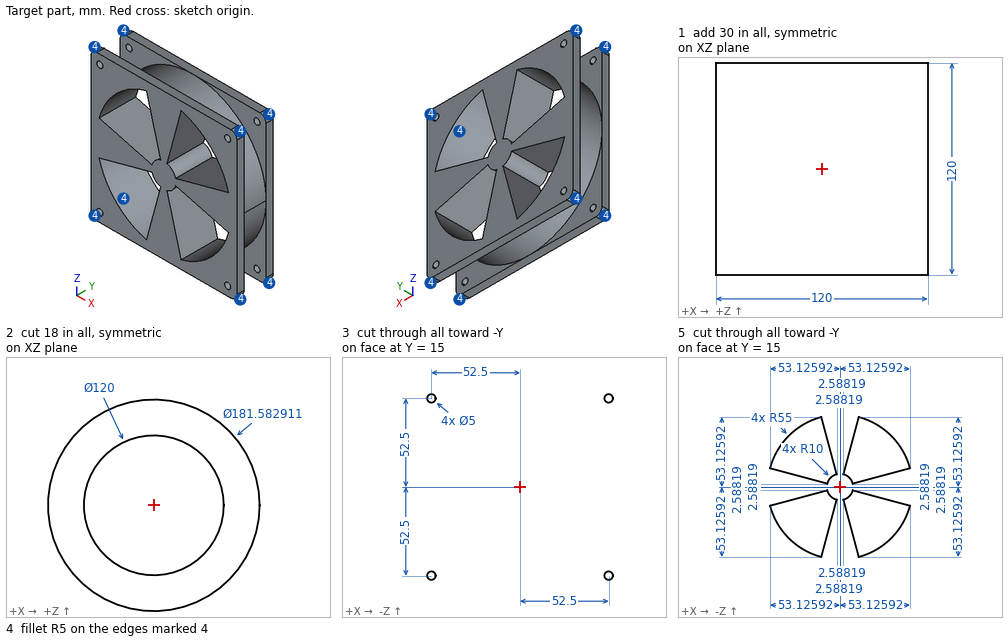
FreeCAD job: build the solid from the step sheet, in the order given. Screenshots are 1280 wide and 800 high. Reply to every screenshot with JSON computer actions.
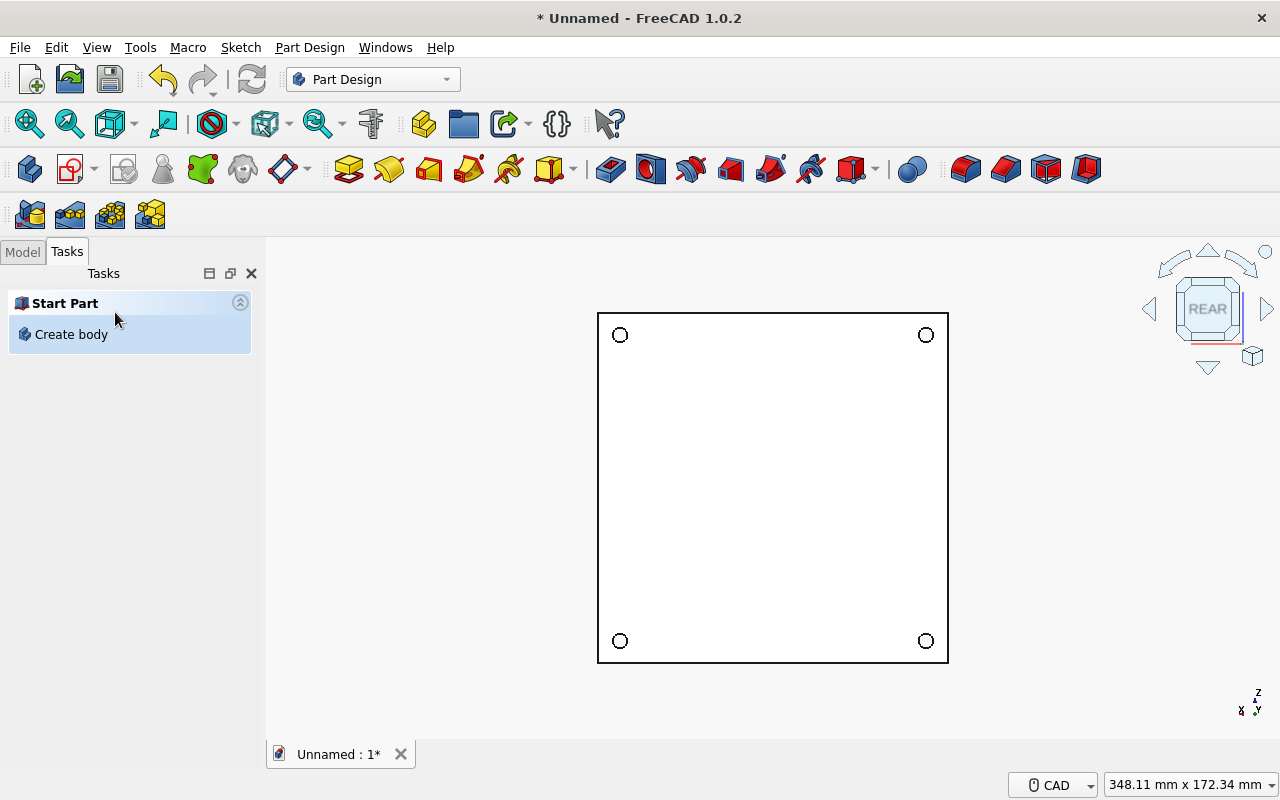
{"action": "scroll", "coordinate": [598, 312], "scroll_direction": "up", "scroll_amount": 5}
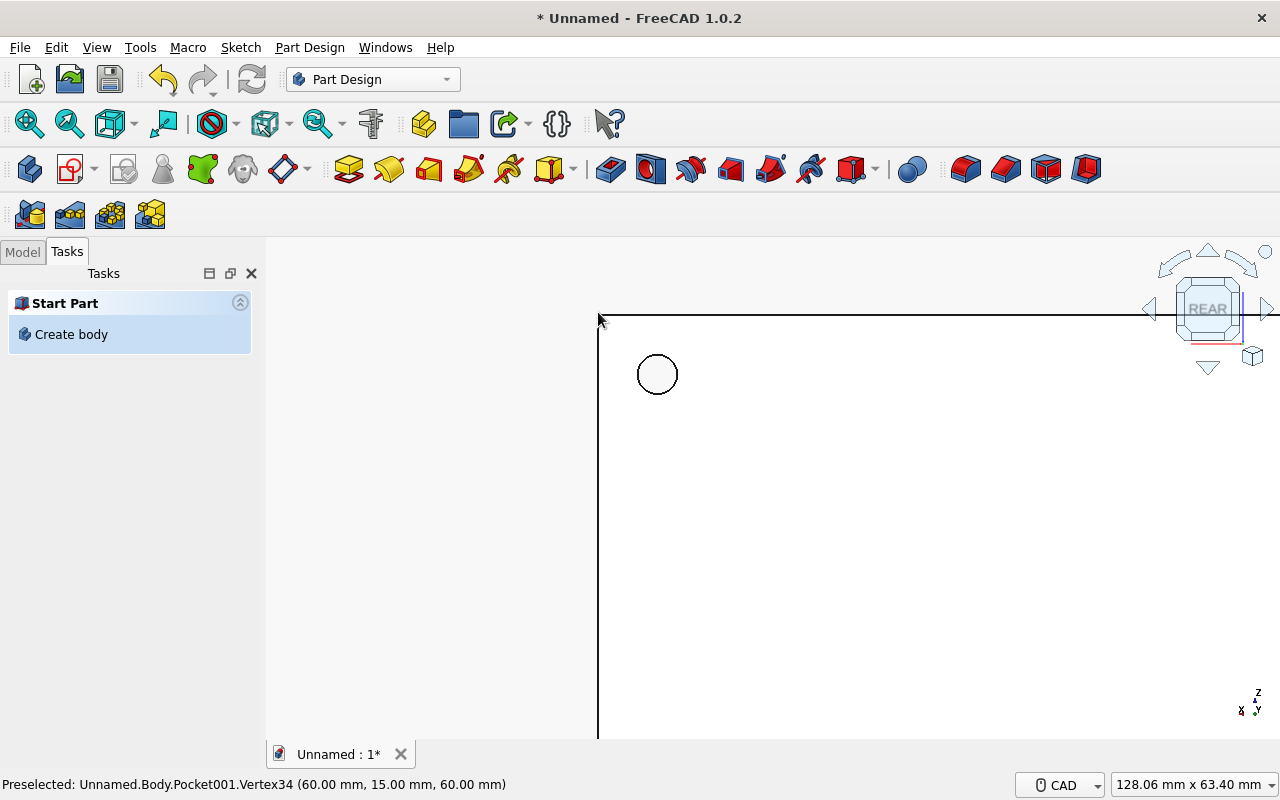
{"action": "left_click", "coordinate": [30, 124]}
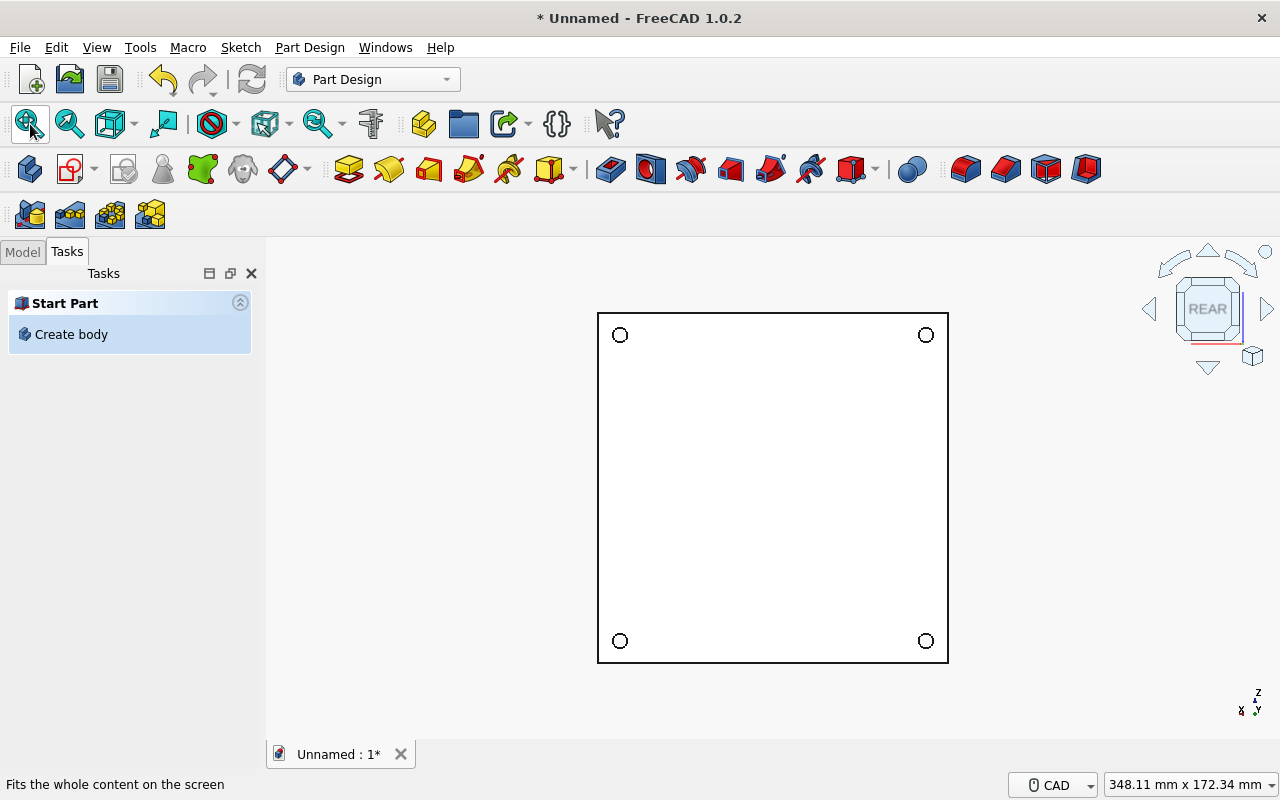
{"action": "key", "text": "0"}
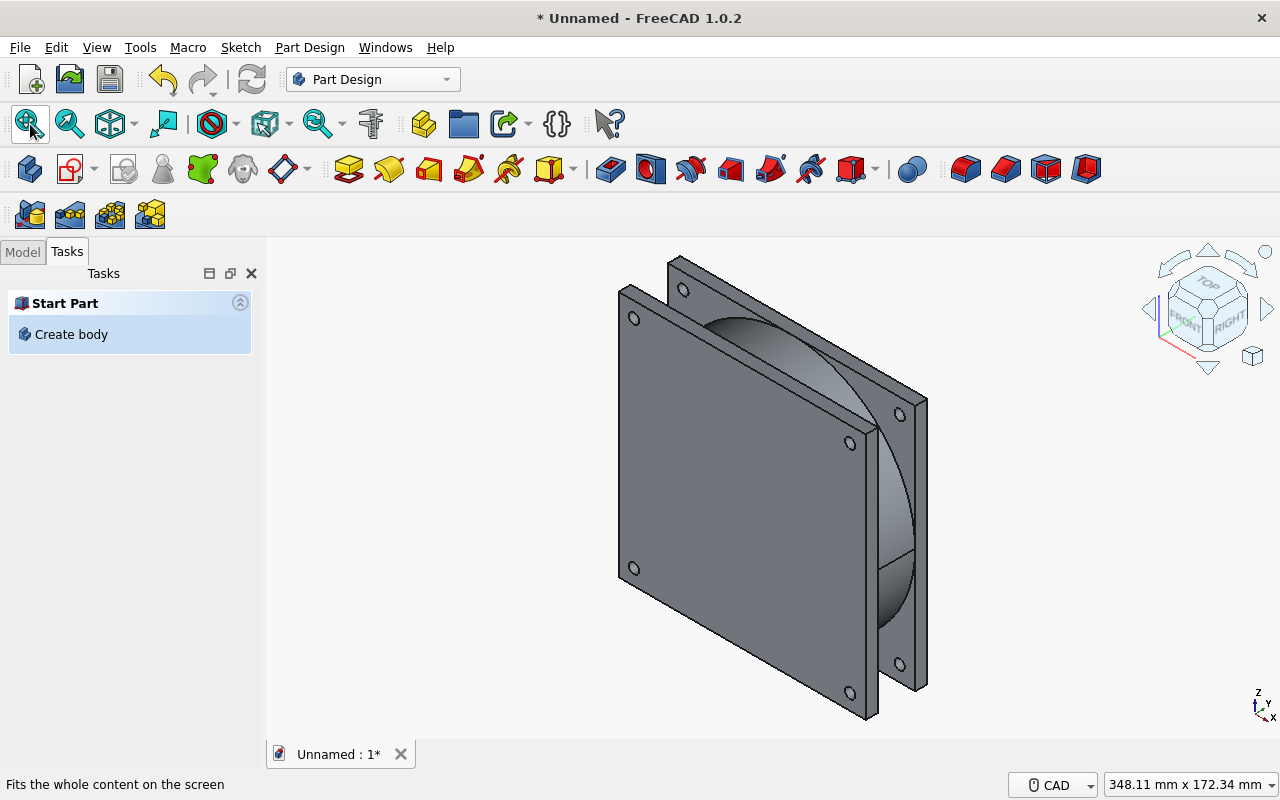
{"action": "left_click", "coordinate": [872, 430]}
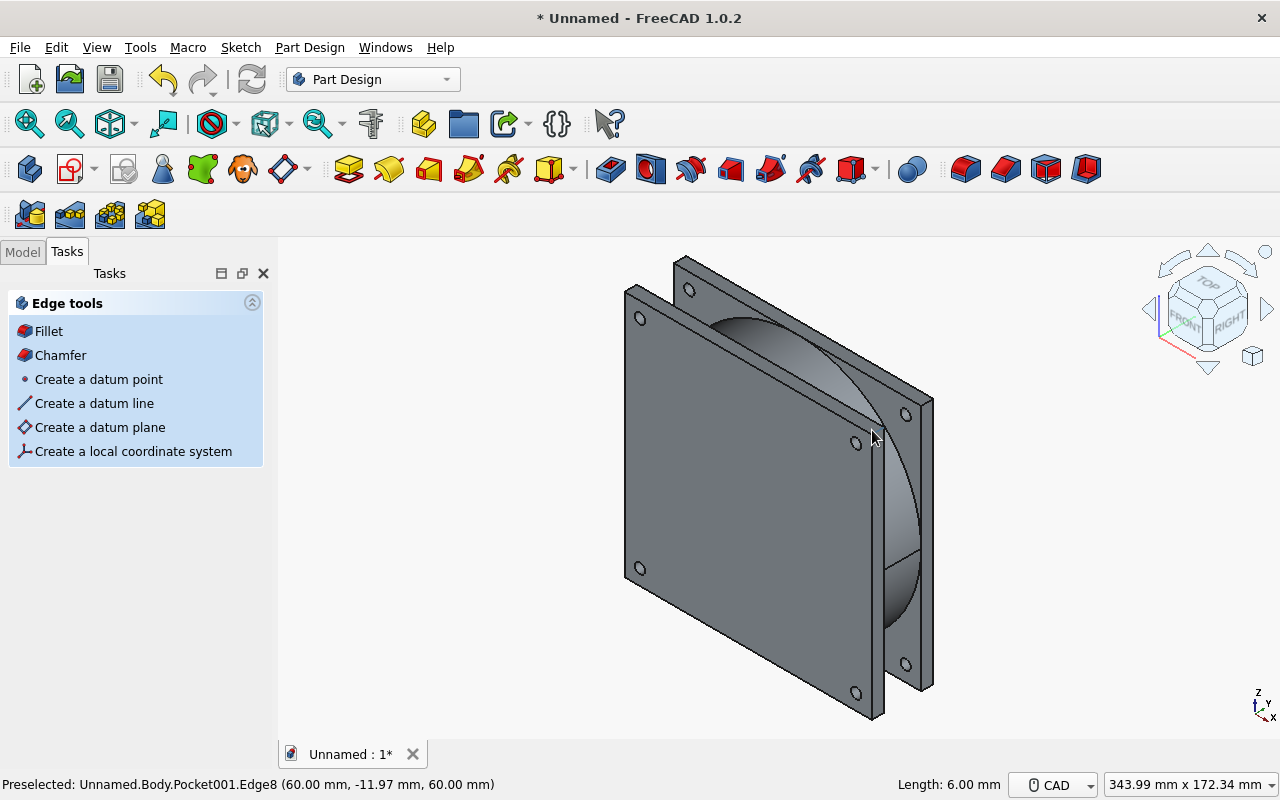
{"action": "left_click", "coordinate": [927, 401], "text": "ctrl"}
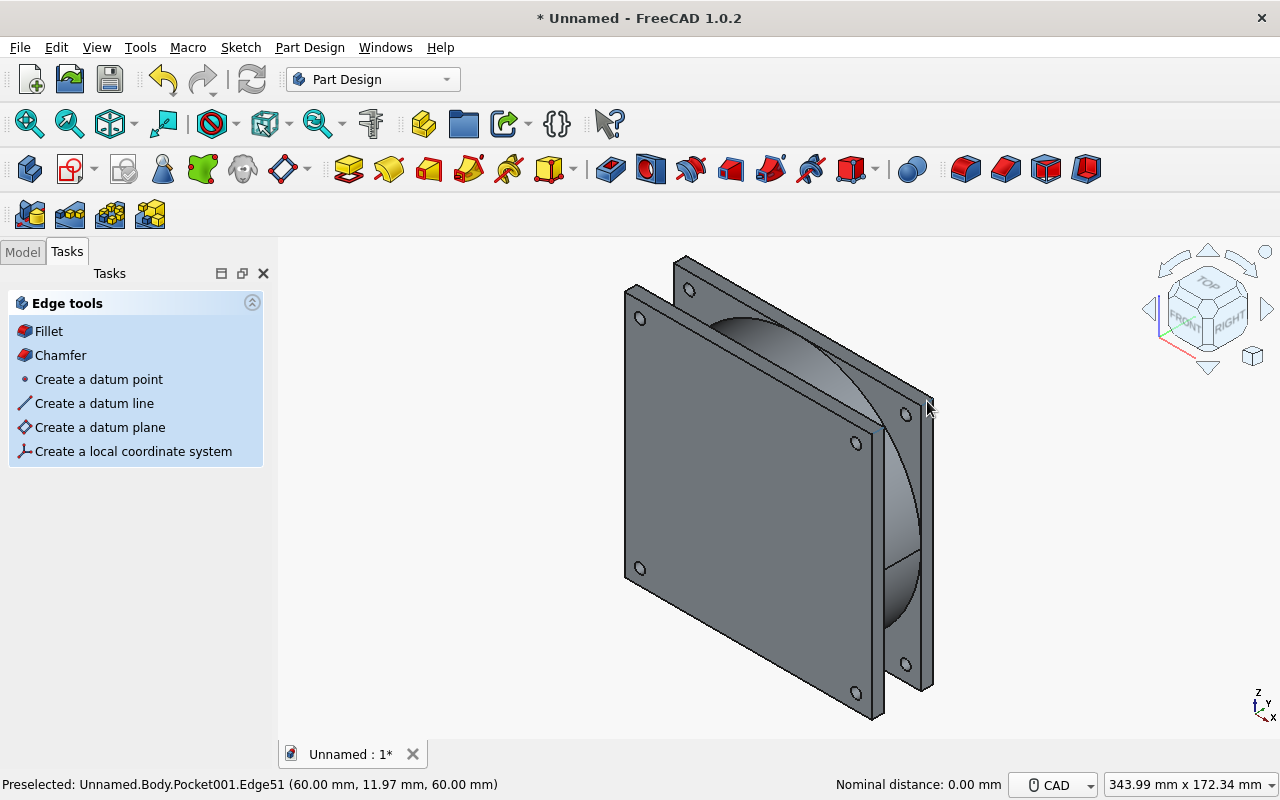
{"action": "scroll", "coordinate": [631, 287], "scroll_direction": "up", "scroll_amount": 5}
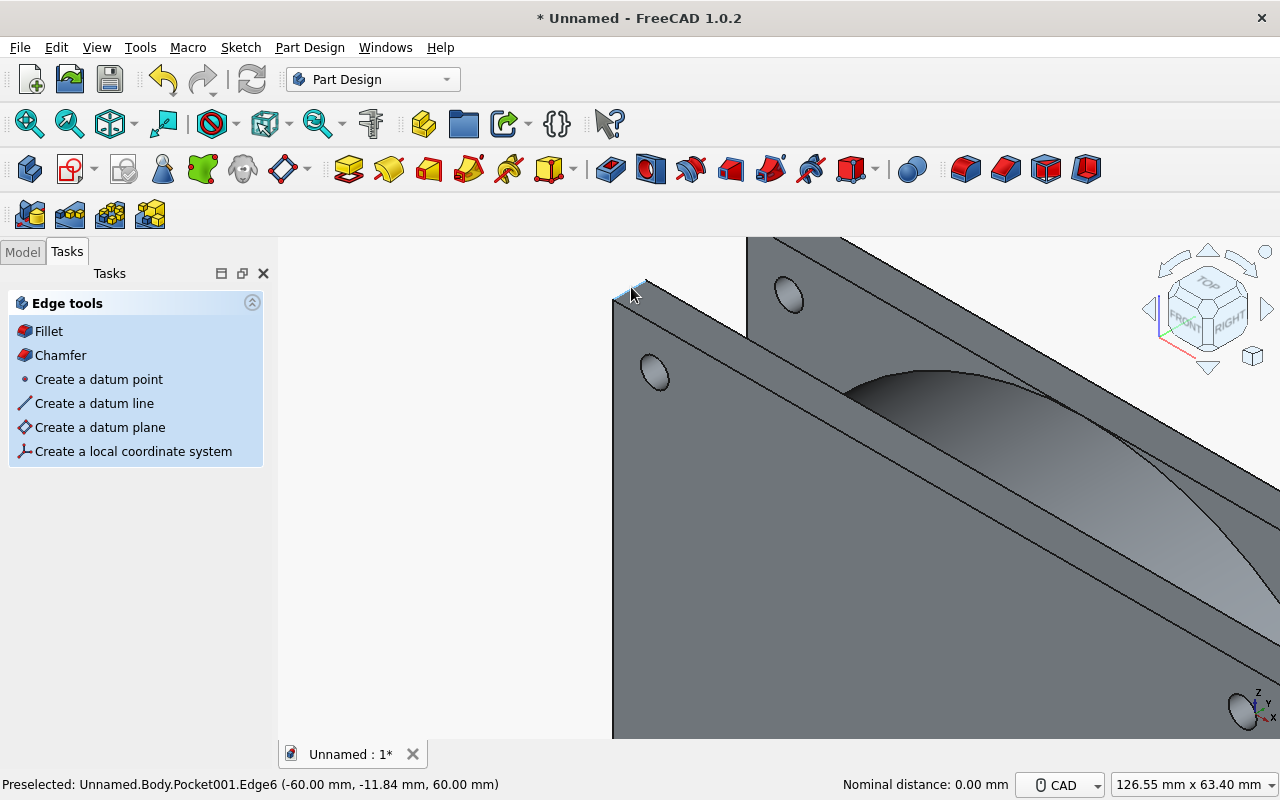
{"action": "left_click", "coordinate": [30, 124]}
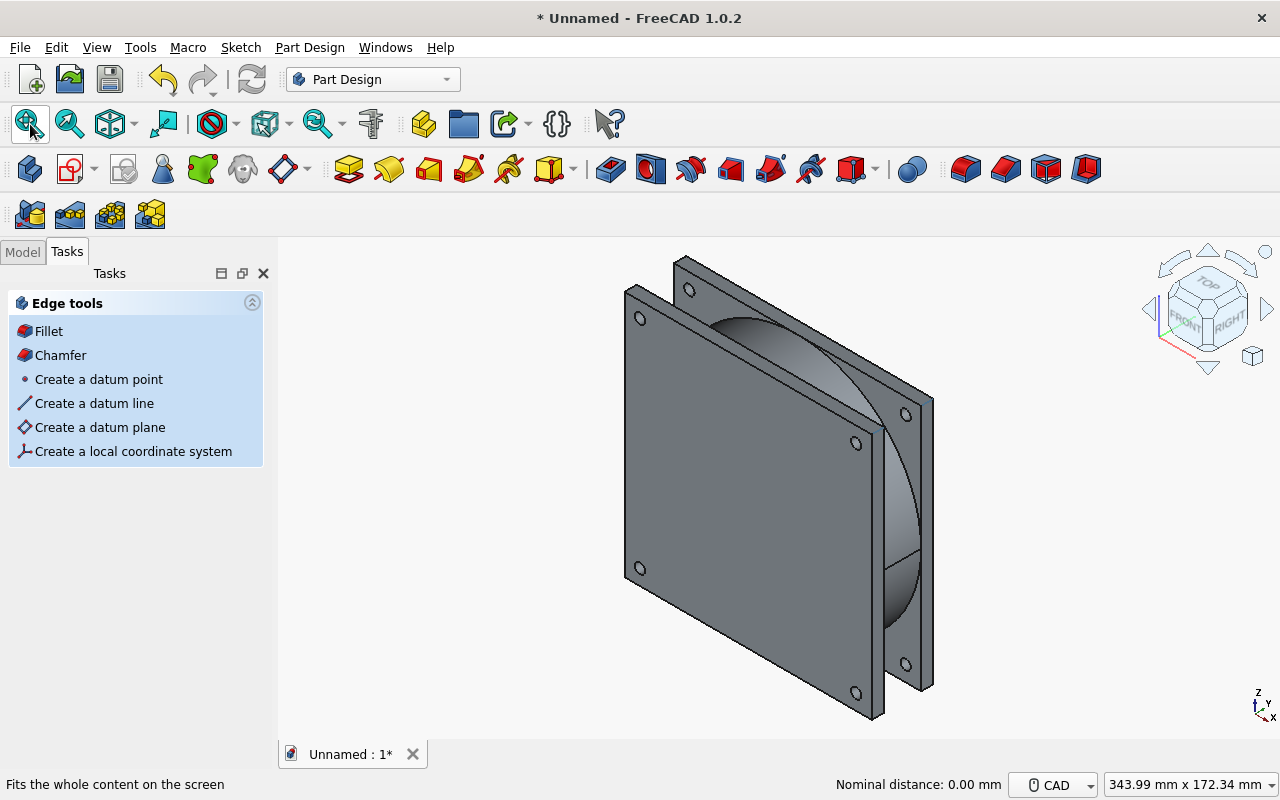
{"action": "key", "text": "2"}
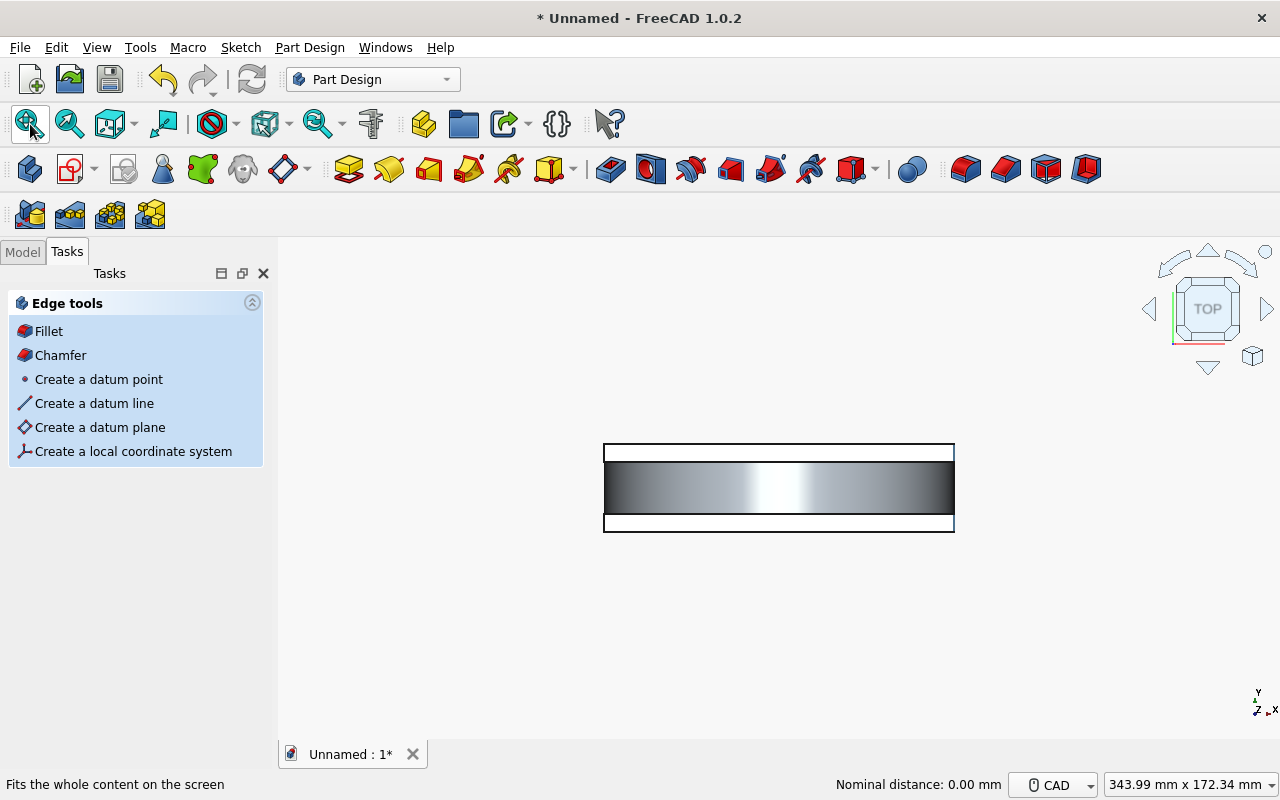
{"action": "left_click", "coordinate": [30, 124]}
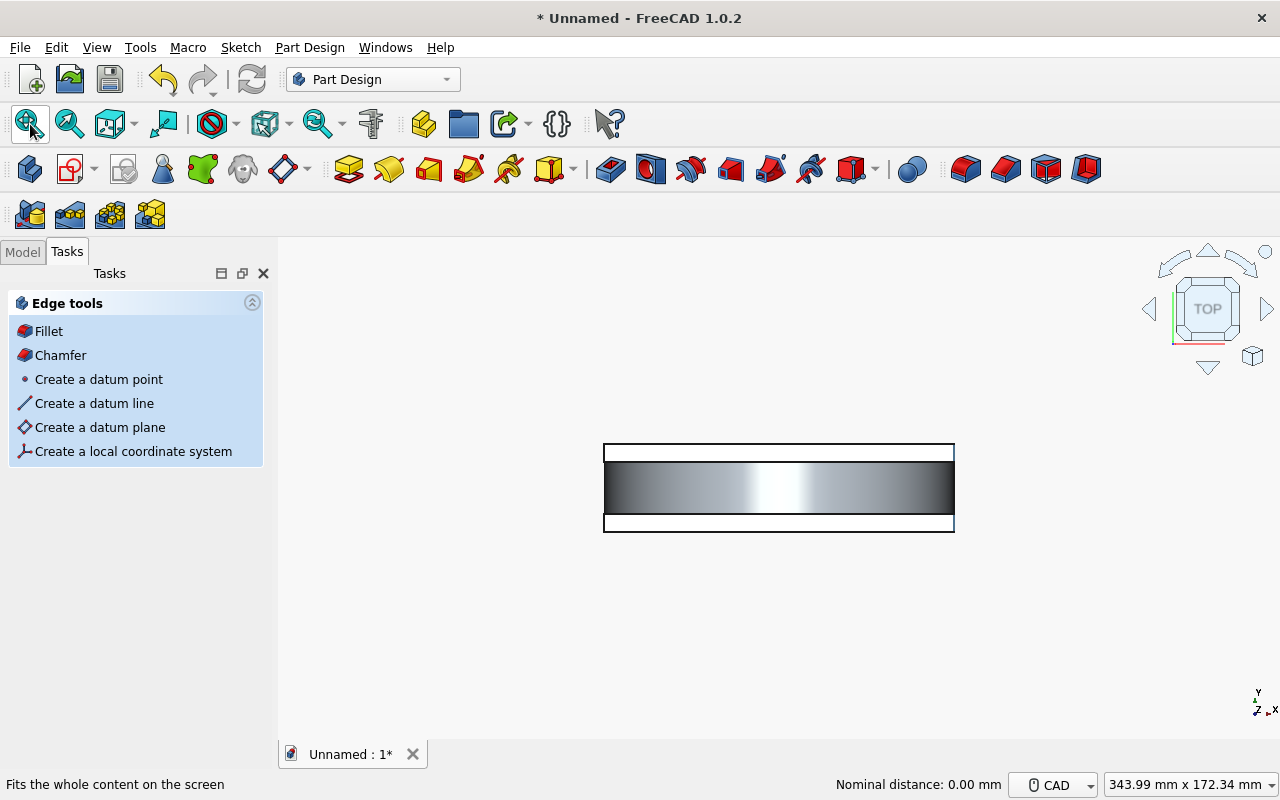
{"action": "left_click", "coordinate": [604, 522], "text": "ctrl"}